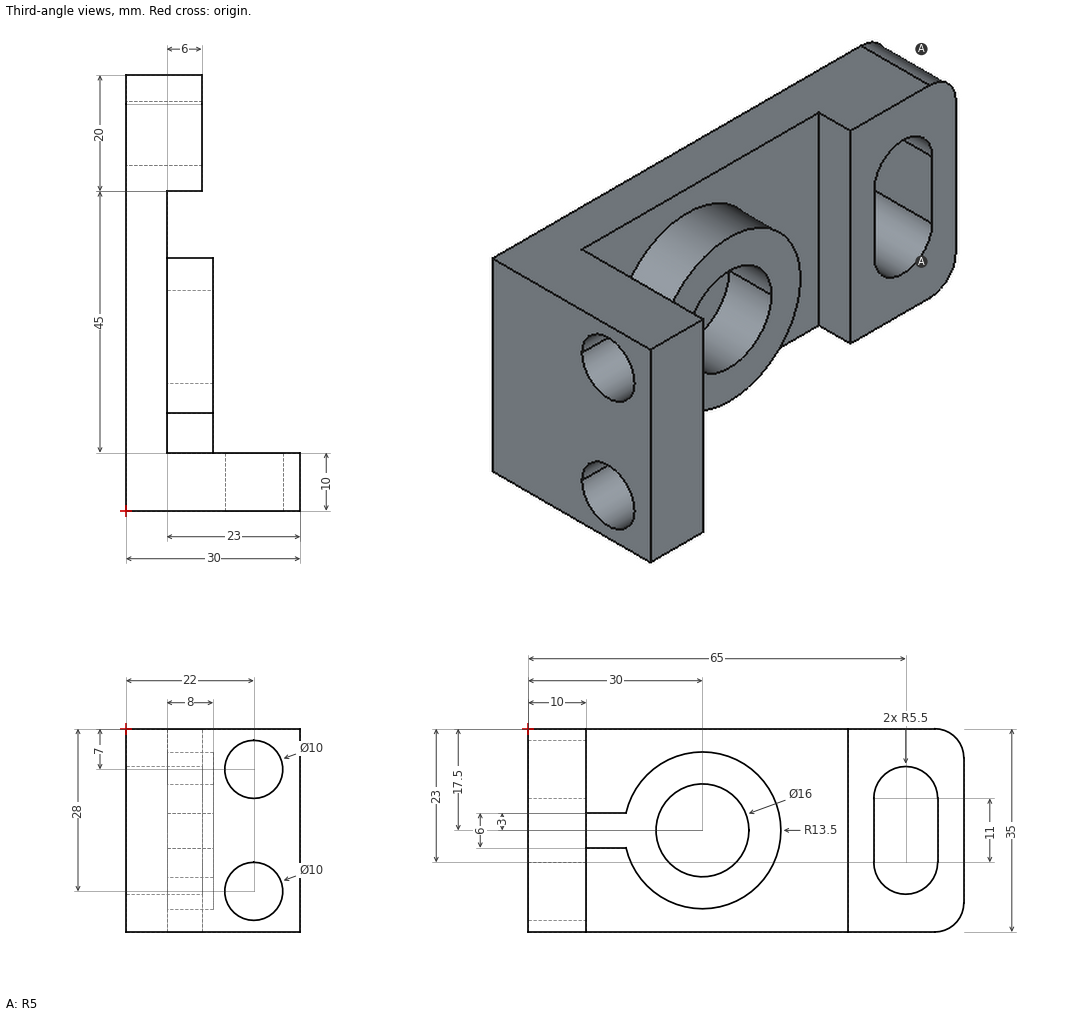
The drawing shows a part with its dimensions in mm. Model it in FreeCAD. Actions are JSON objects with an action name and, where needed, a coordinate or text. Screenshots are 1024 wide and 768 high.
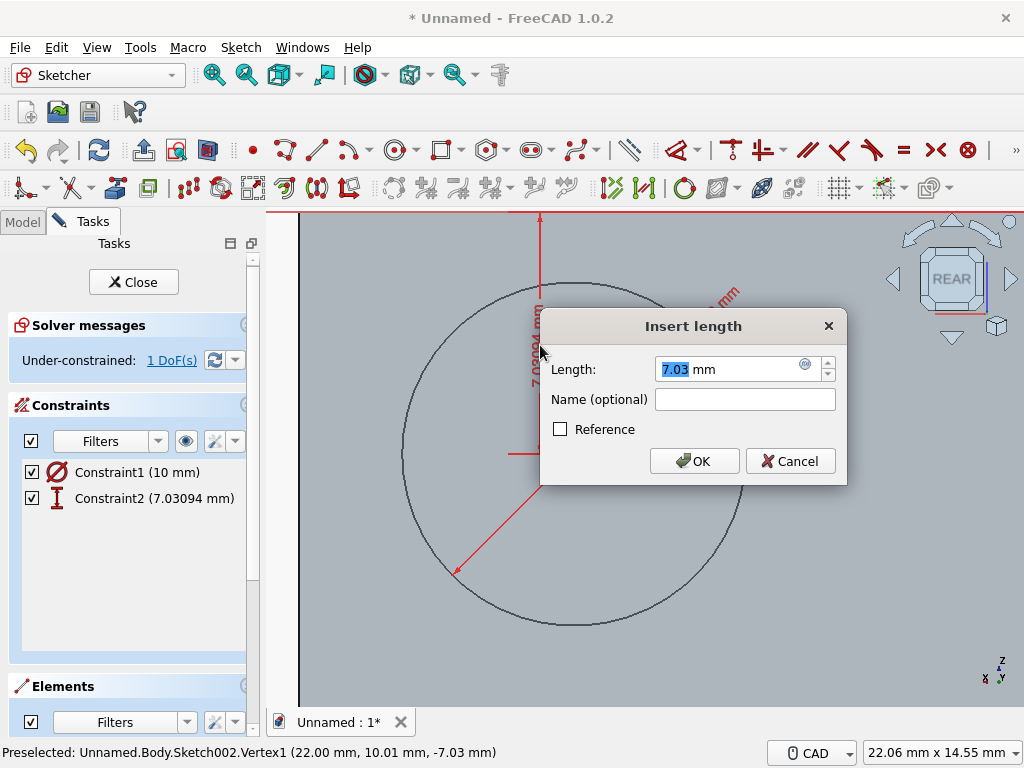
{"action": "type", "text": "7"}
{"action": "key", "text": "Return"}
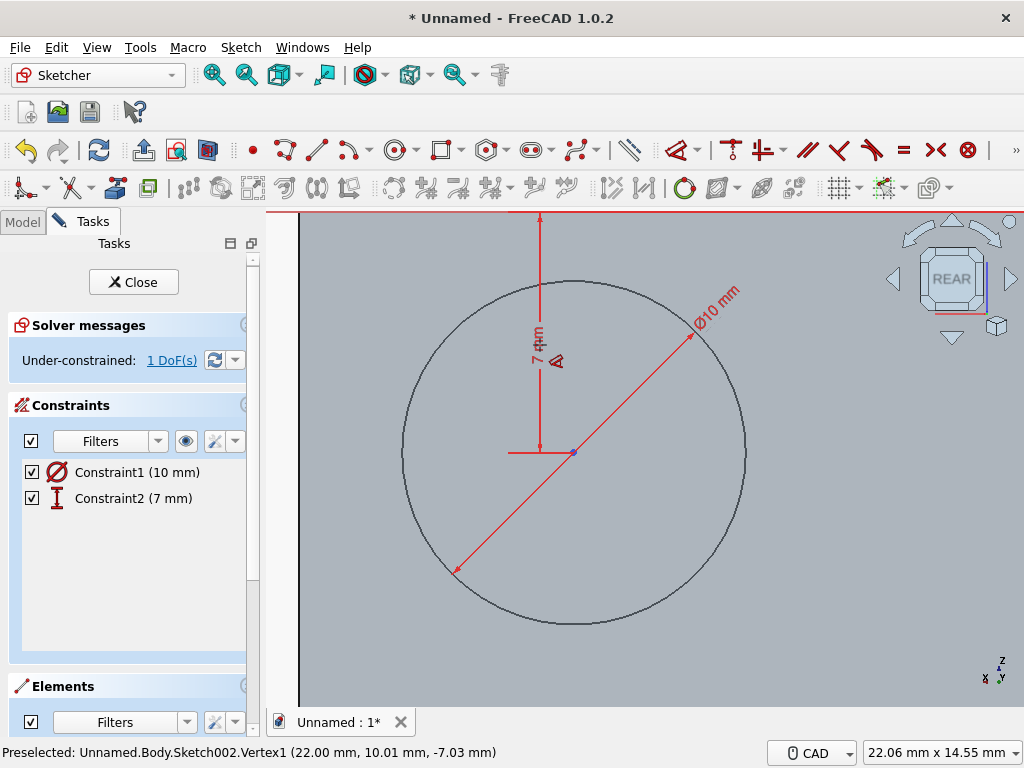
{"action": "left_click", "coordinate": [574, 453]}
{"action": "left_click", "coordinate": [716, 487]}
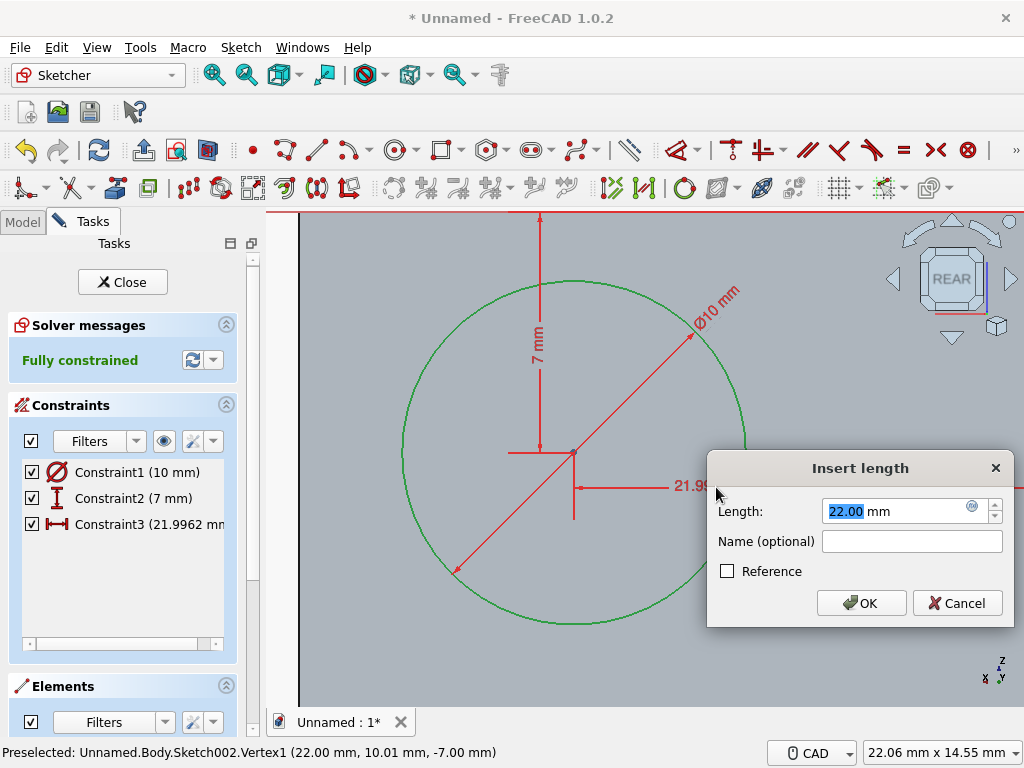
{"action": "type", "text": "22"}
{"action": "key", "text": "Return"}
{"action": "key", "text": "Escape"}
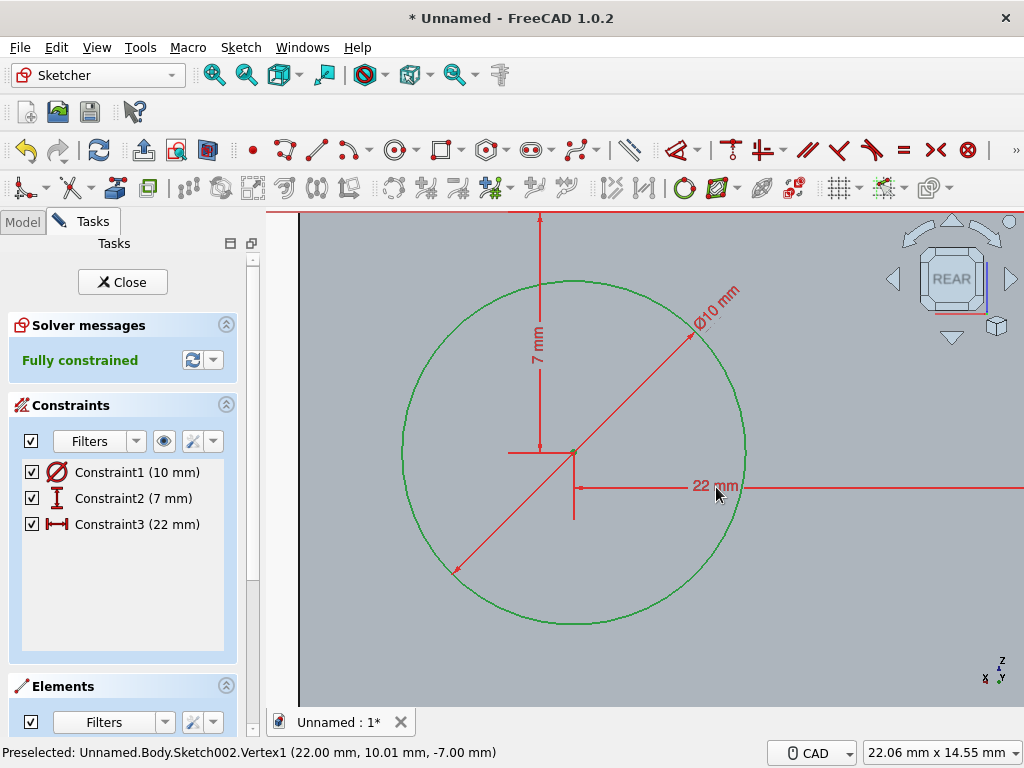
{"action": "left_click", "coordinate": [123, 282]}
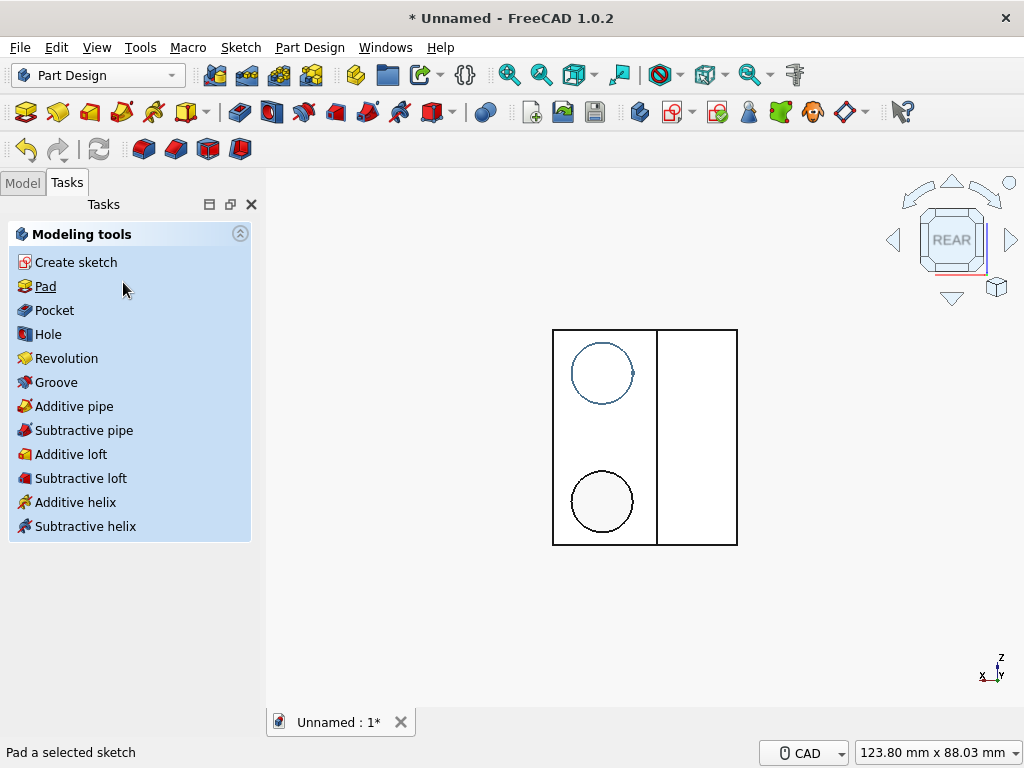
{"action": "left_click", "coordinate": [240, 112]}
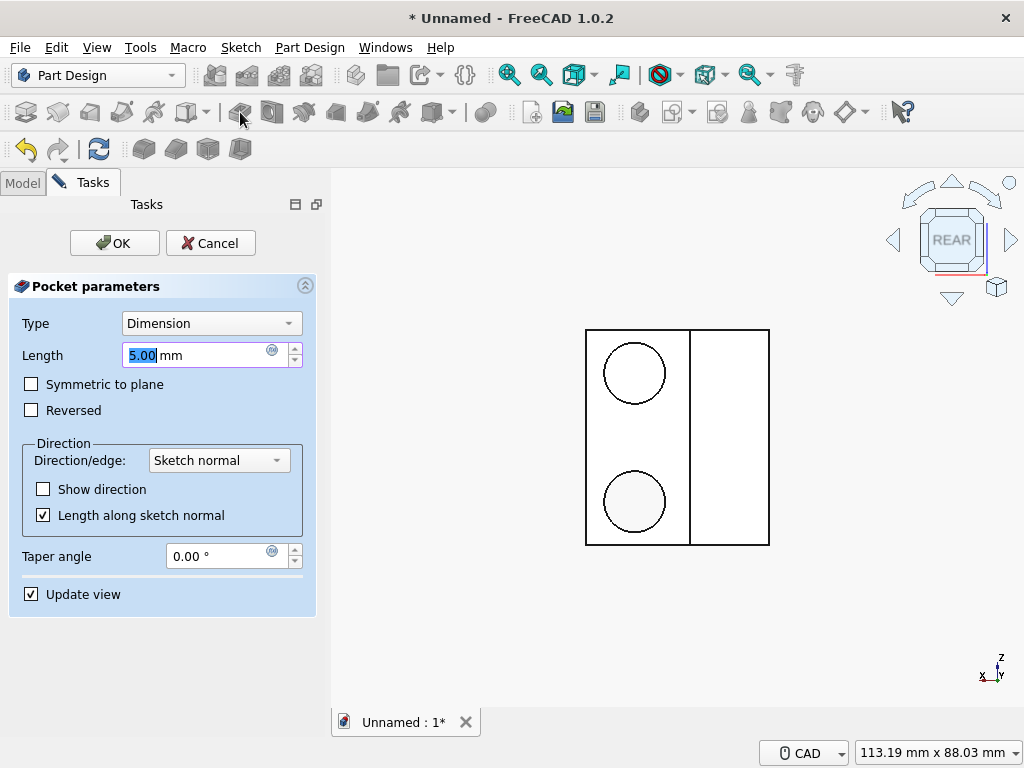
{"action": "left_click", "coordinate": [212, 324]}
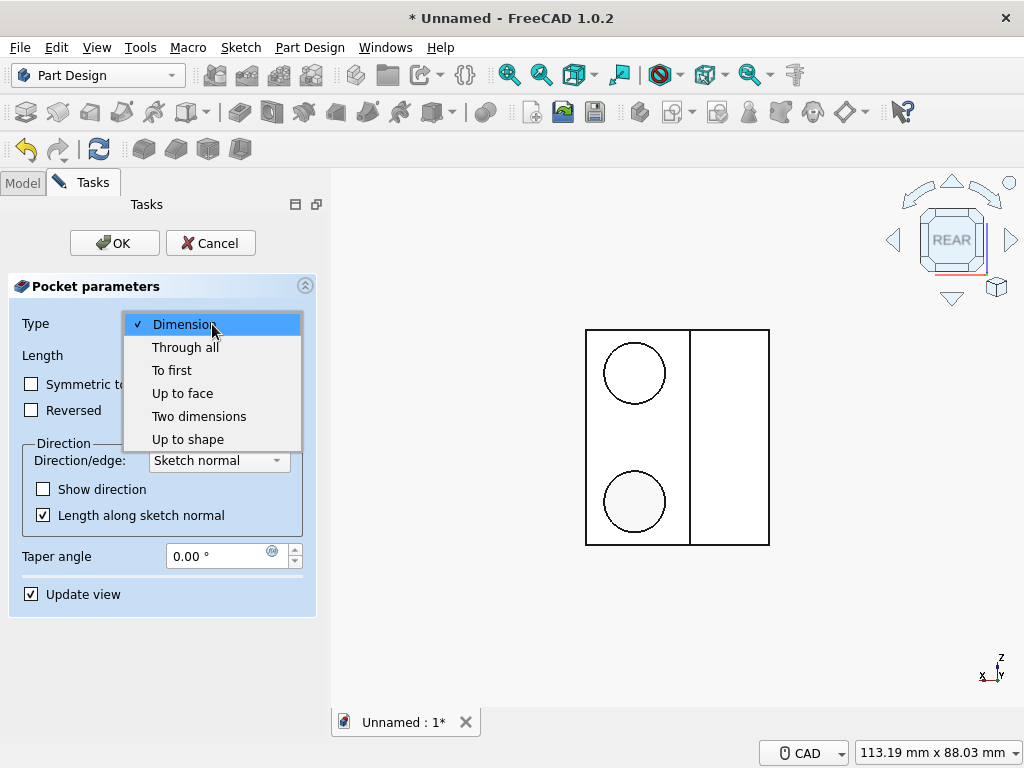
{"action": "left_click", "coordinate": [212, 370]}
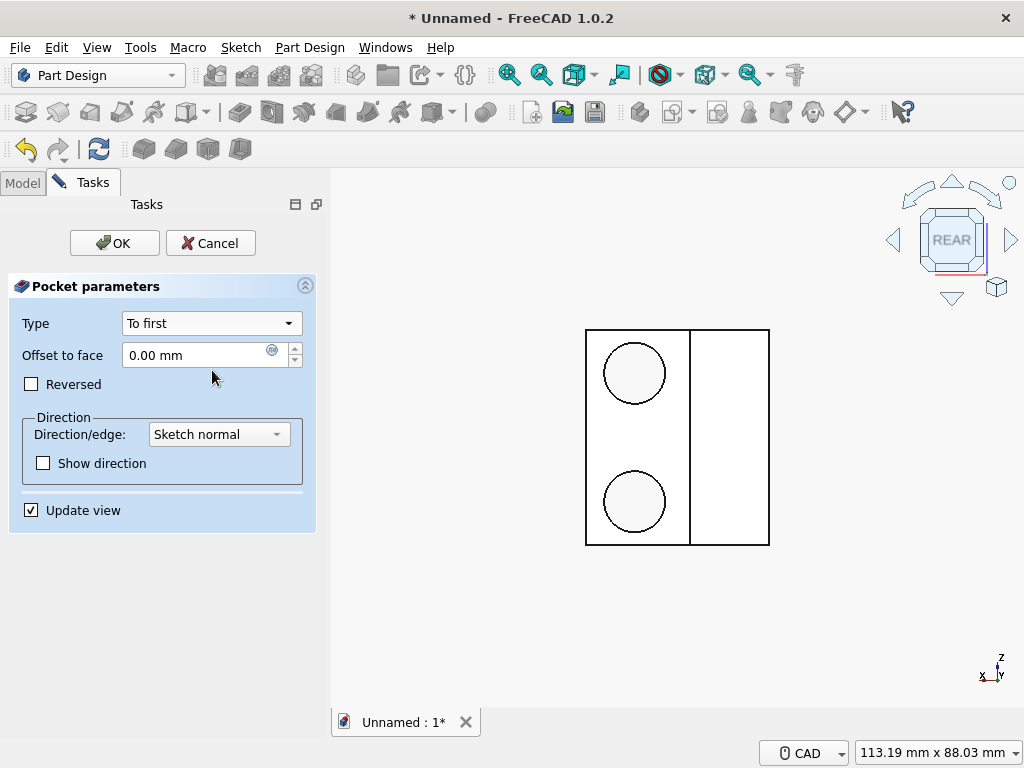
{"action": "left_click", "coordinate": [115, 243]}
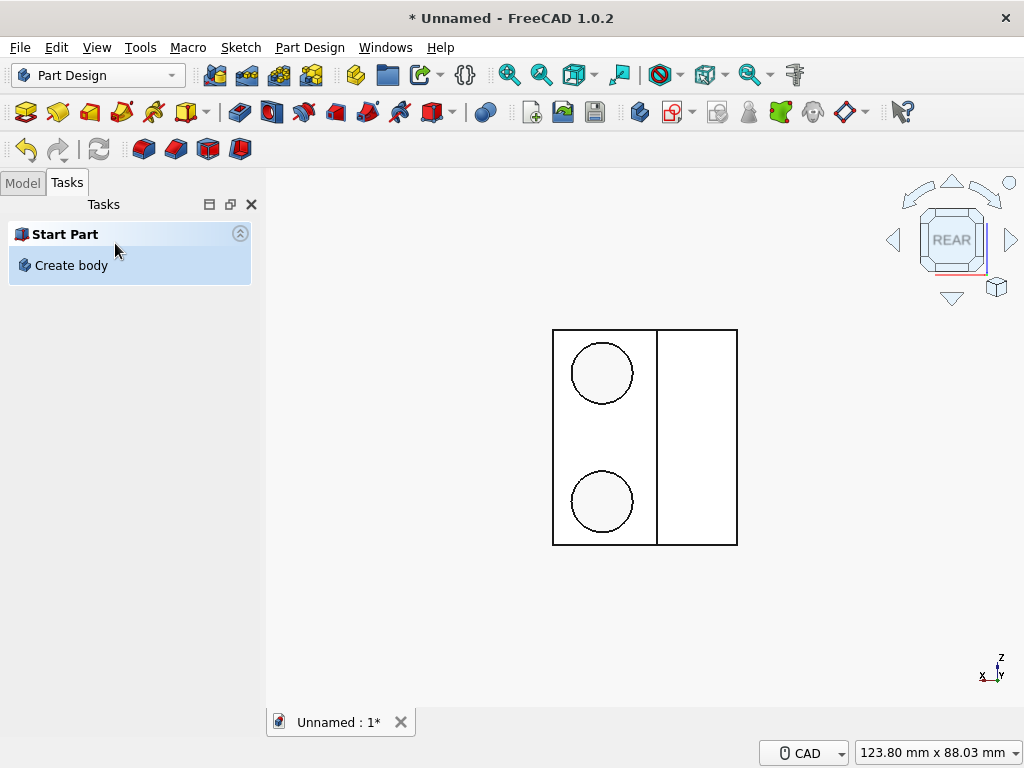
{"action": "left_click", "coordinate": [510, 76]}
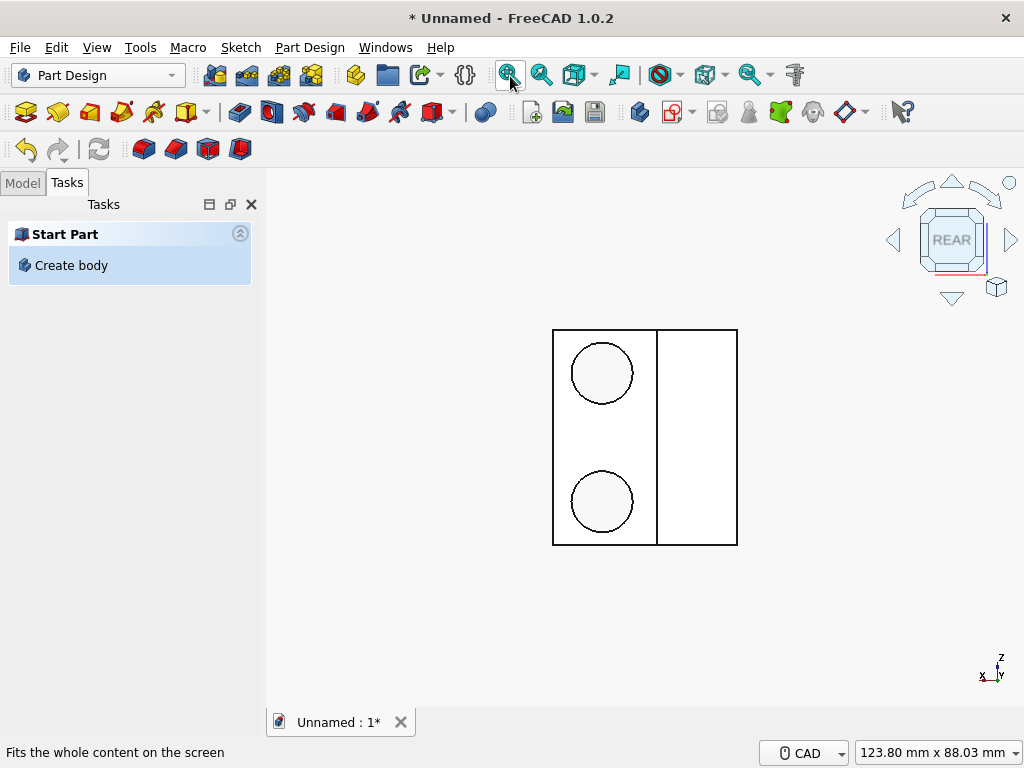
{"action": "key", "text": "0"}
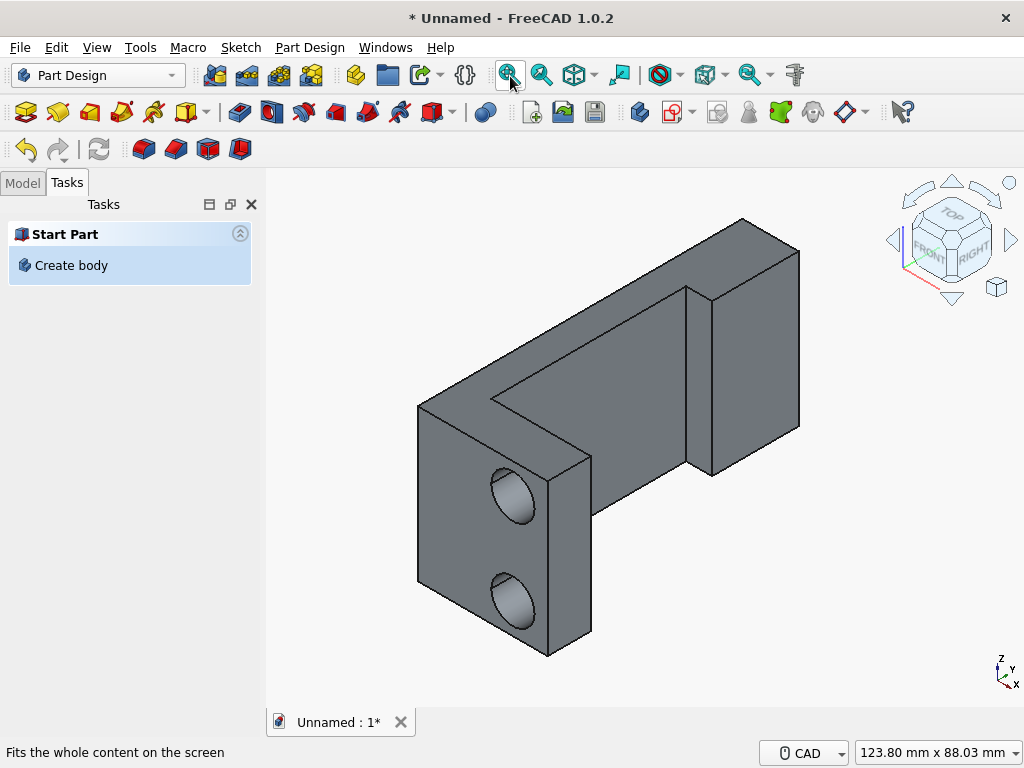
{"action": "left_click", "coordinate": [589, 429]}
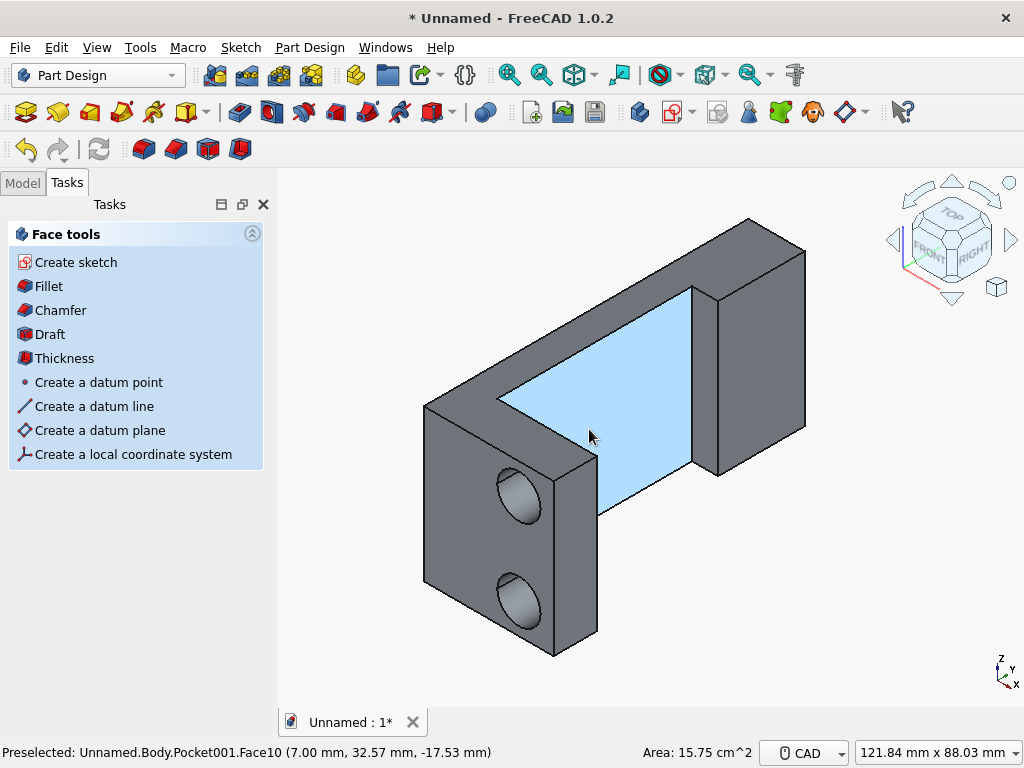
{"action": "left_click", "coordinate": [672, 112]}